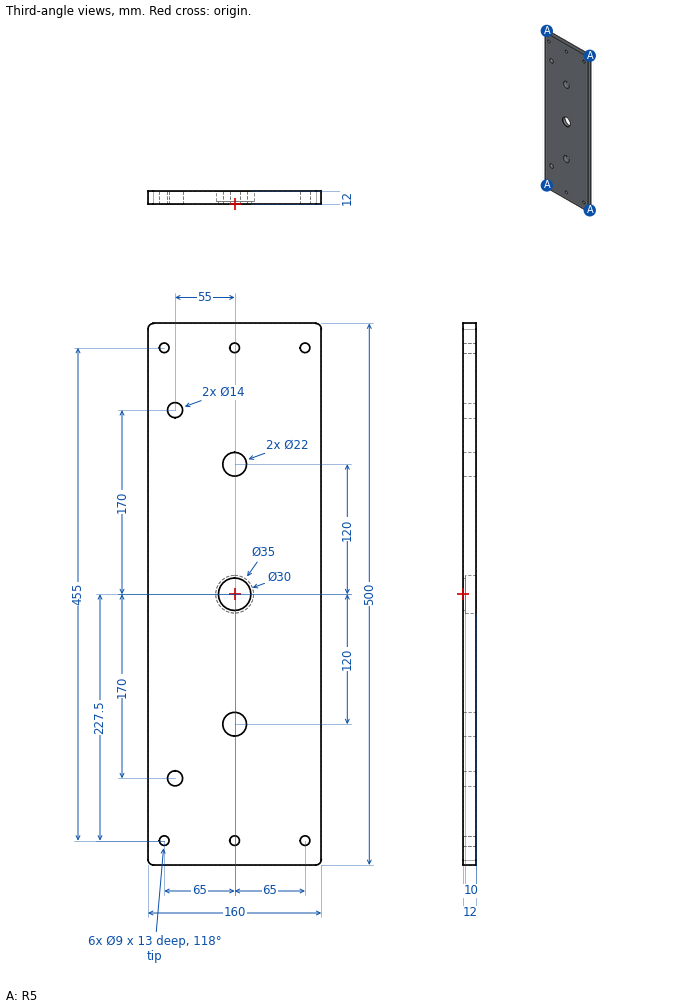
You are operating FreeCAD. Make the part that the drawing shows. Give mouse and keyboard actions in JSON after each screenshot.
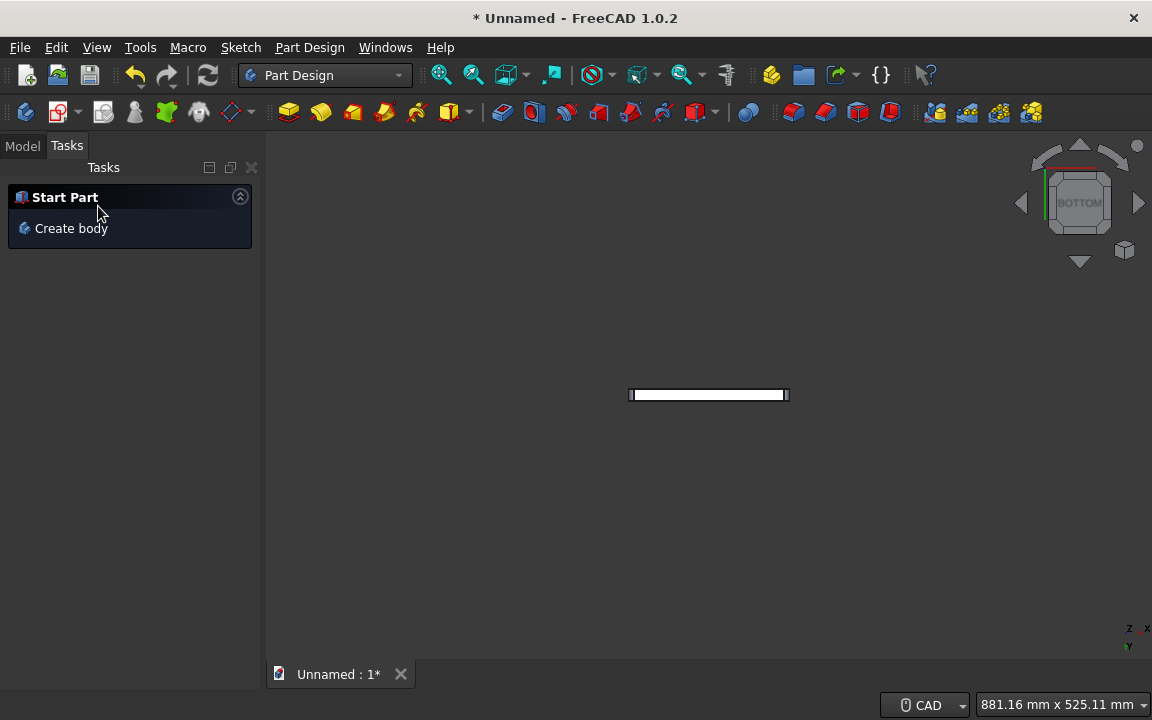
{"action": "left_click", "coordinate": [442, 76]}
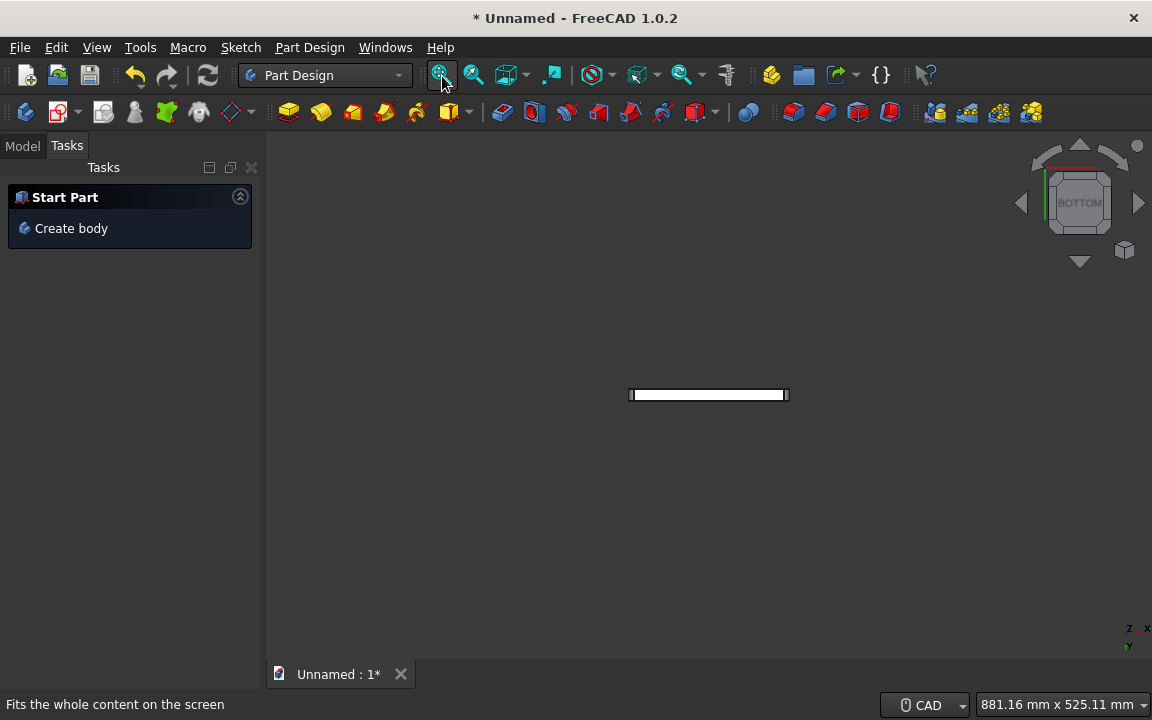
{"action": "left_click", "coordinate": [58, 112]}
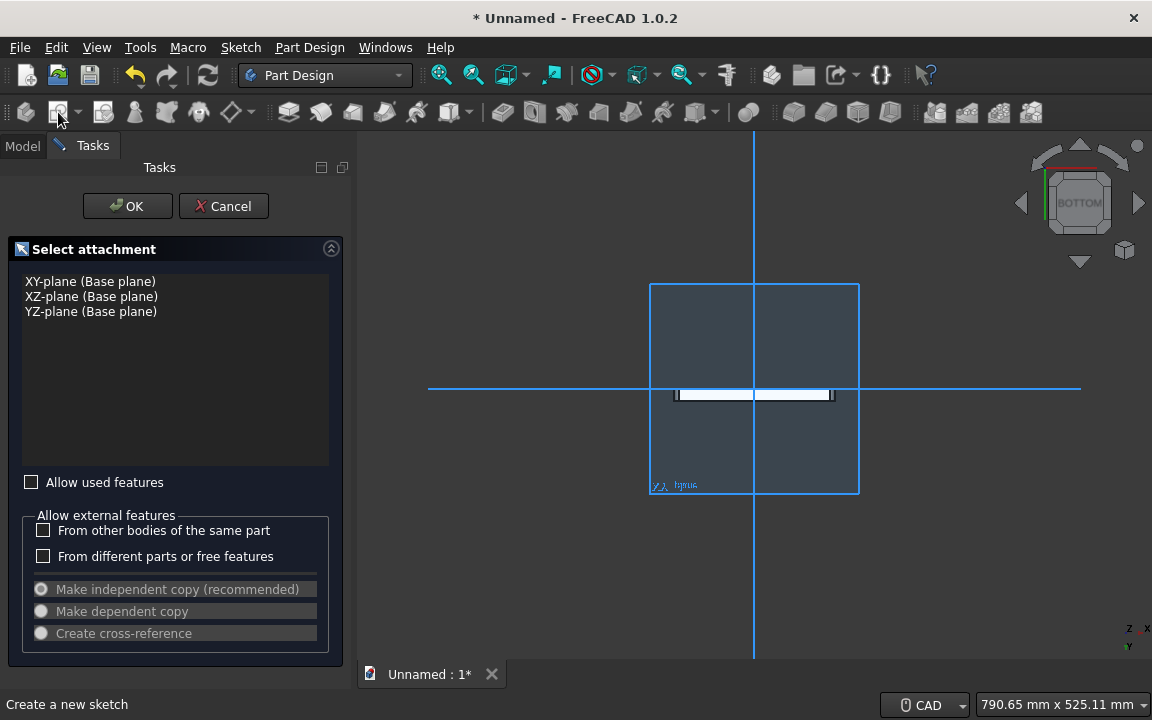
{"action": "left_click", "coordinate": [82, 296]}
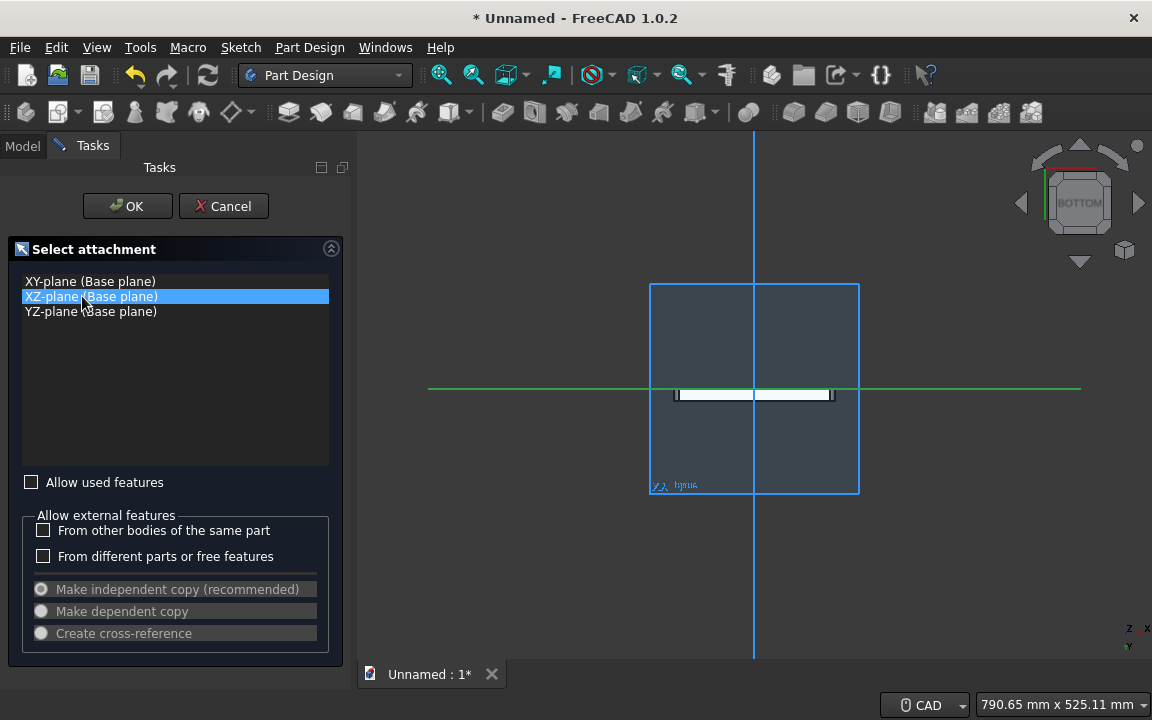
{"action": "left_click", "coordinate": [128, 206]}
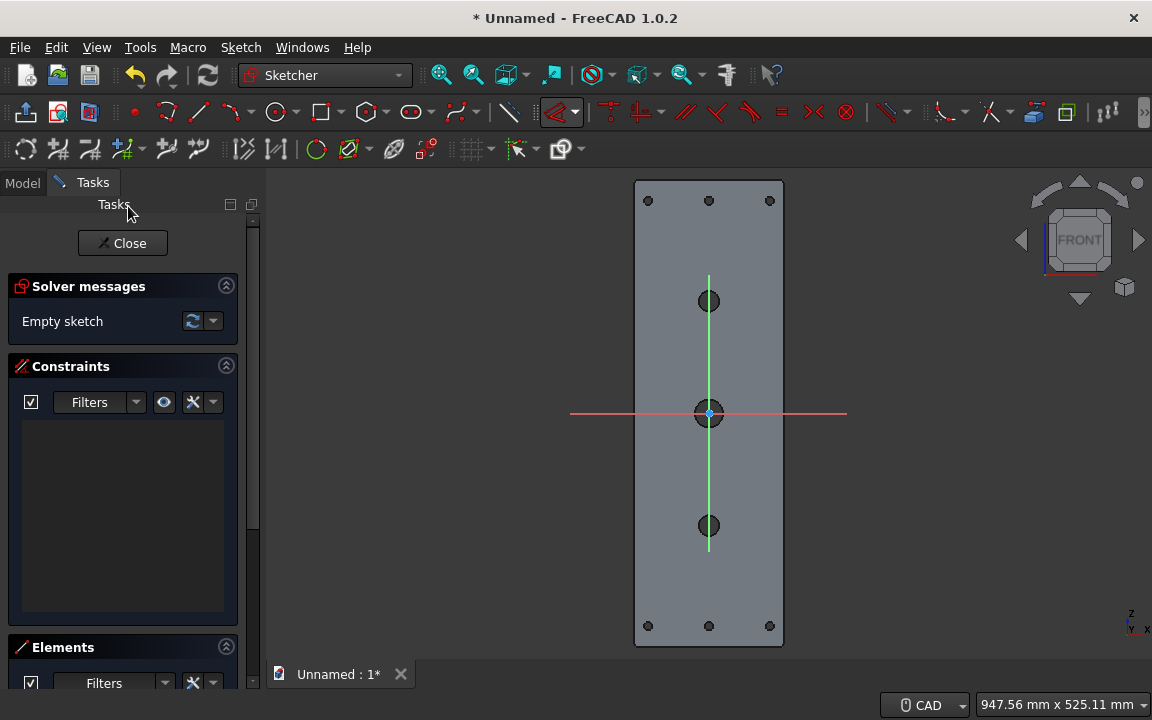
{"action": "left_click", "coordinate": [276, 112]}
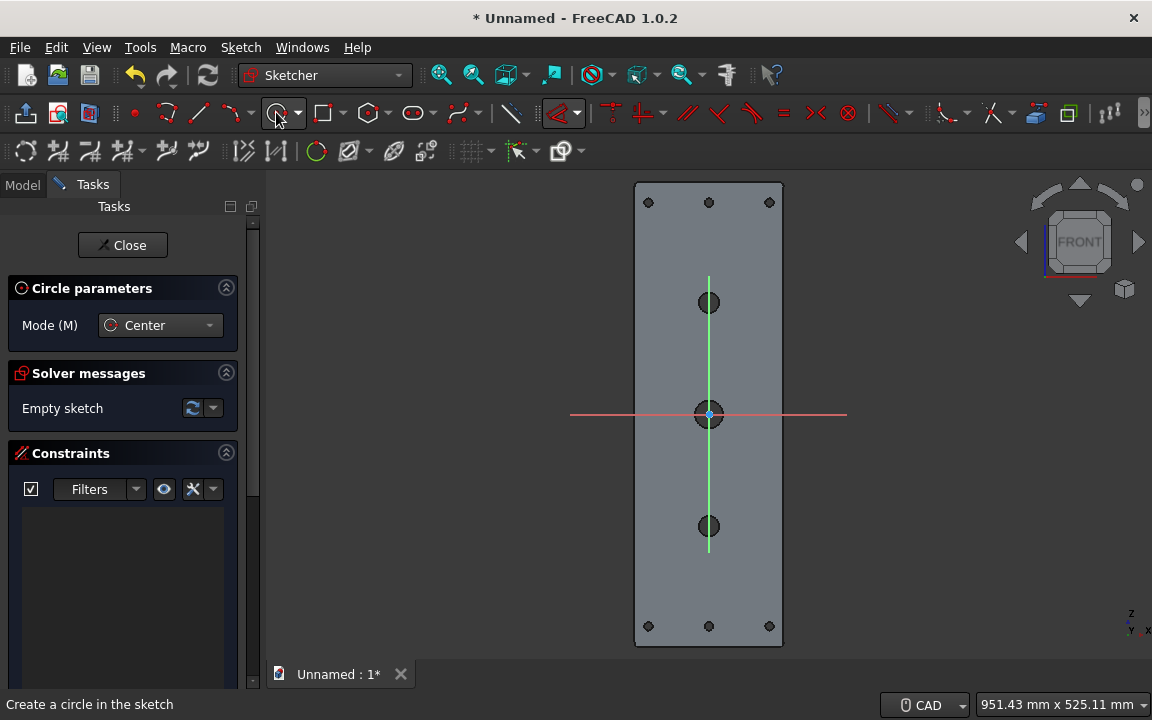
{"action": "scroll", "coordinate": [658, 256], "scroll_direction": "up", "scroll_amount": 7}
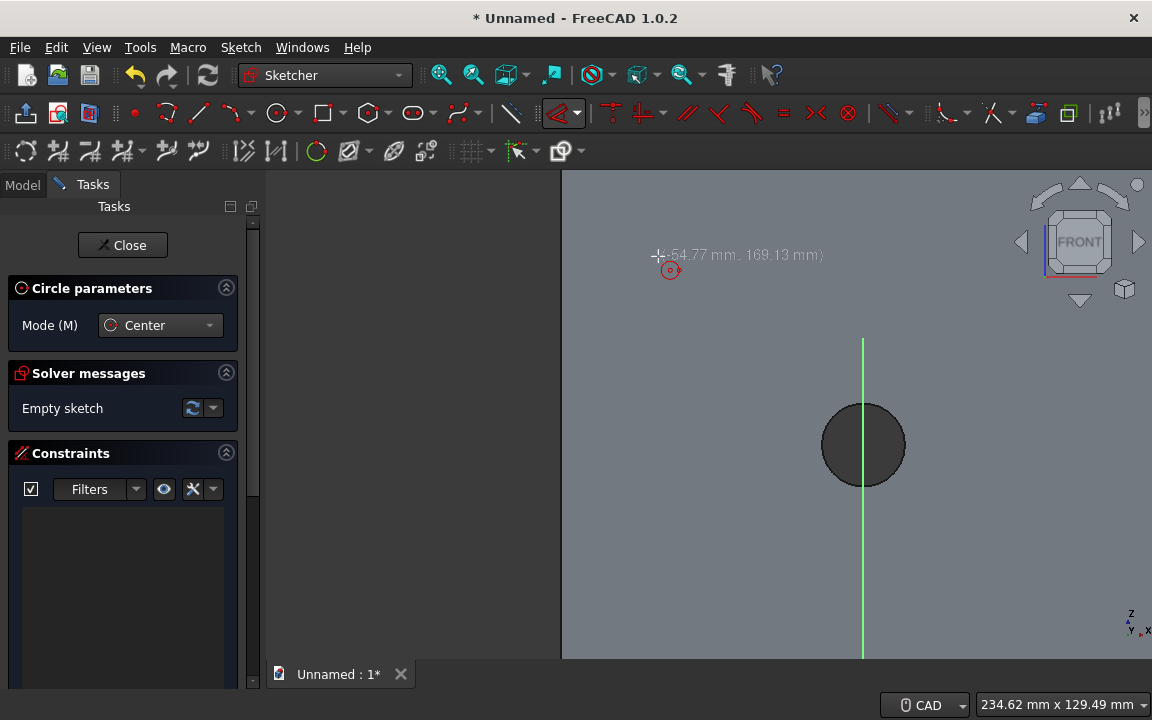
{"action": "scroll", "coordinate": [606, 256], "scroll_direction": "down", "scroll_amount": 7}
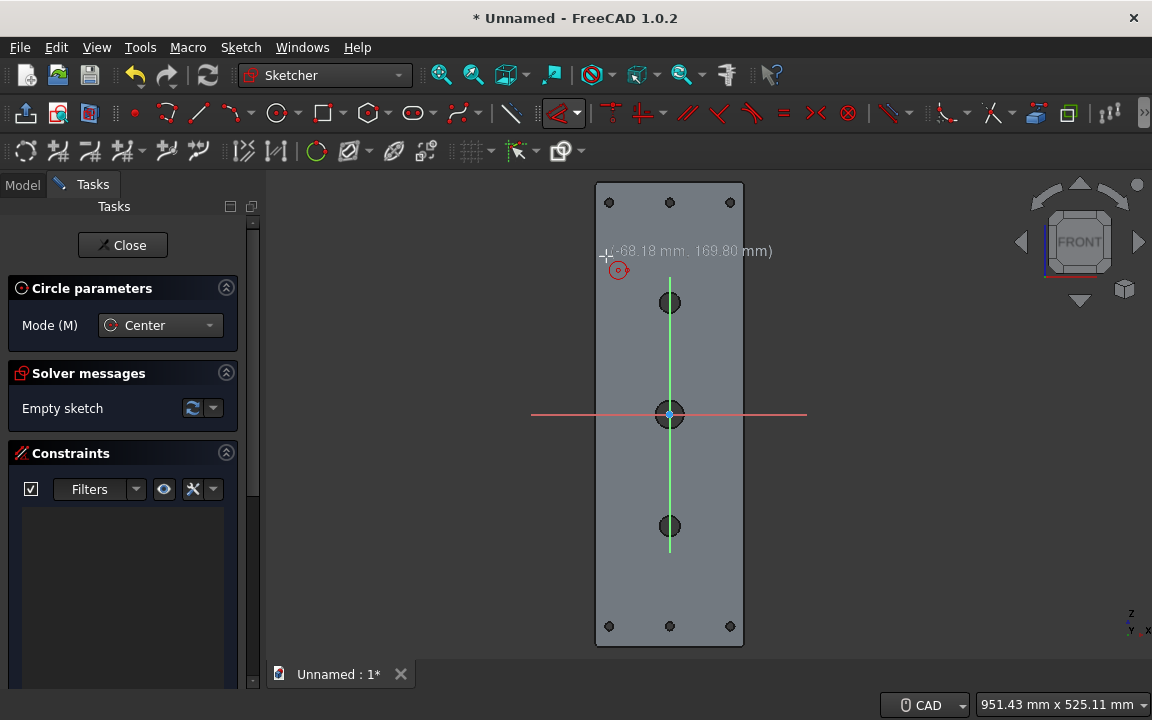
{"action": "left_click", "coordinate": [619, 256]}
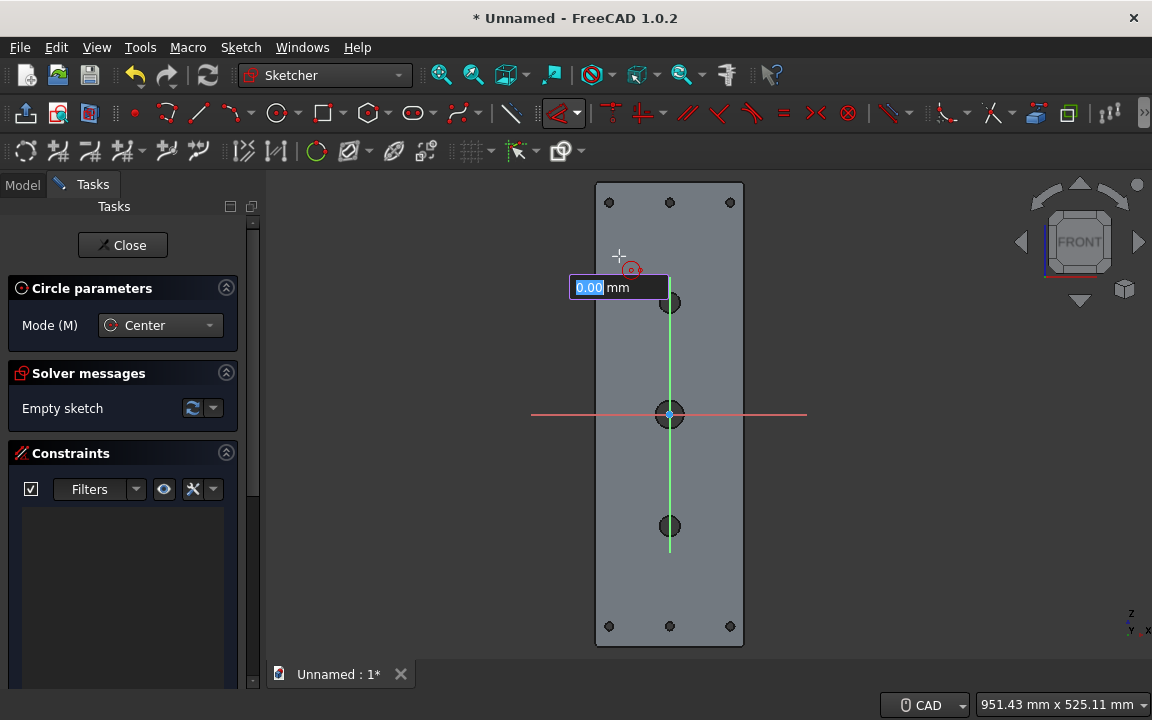
{"action": "scroll", "coordinate": [623, 252], "scroll_direction": "up", "scroll_amount": 5}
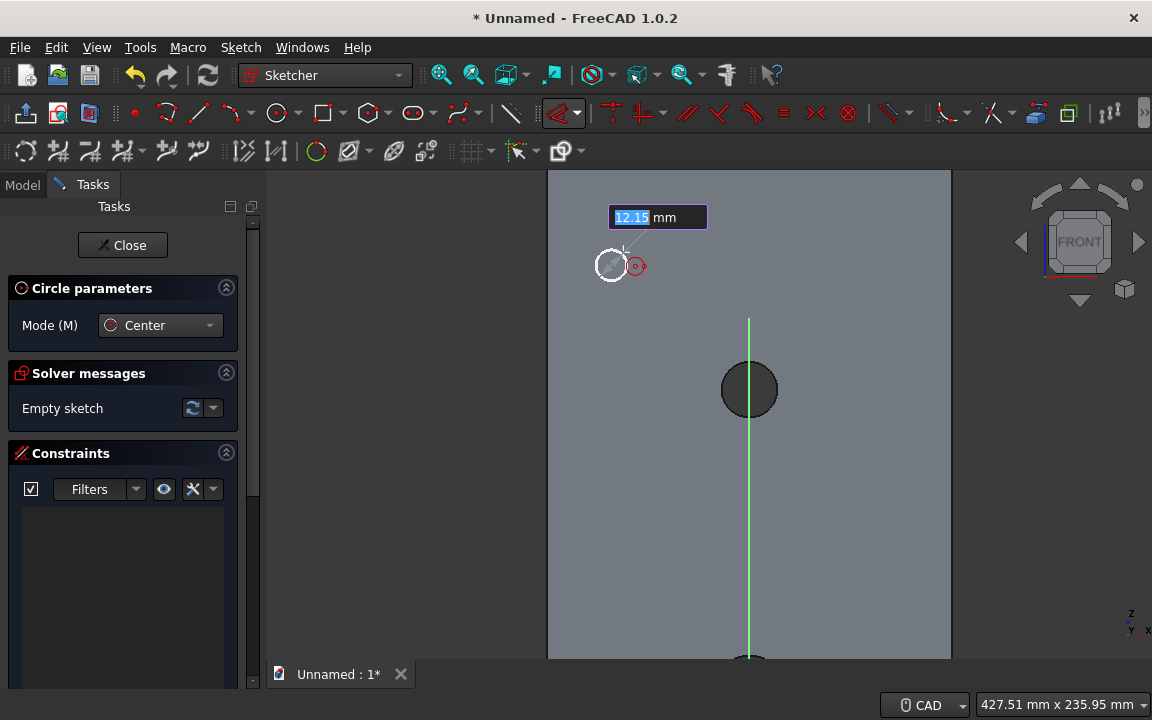
{"action": "left_click", "coordinate": [623, 251]}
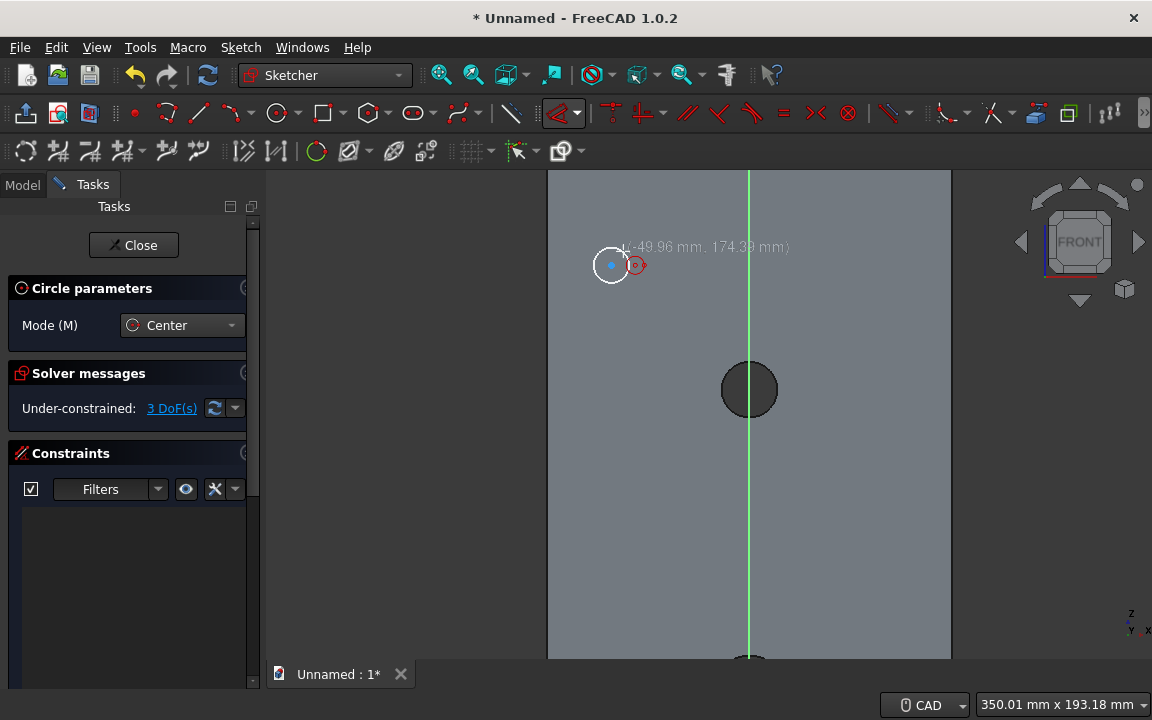
{"action": "scroll", "coordinate": [623, 252], "scroll_direction": "down", "scroll_amount": 5}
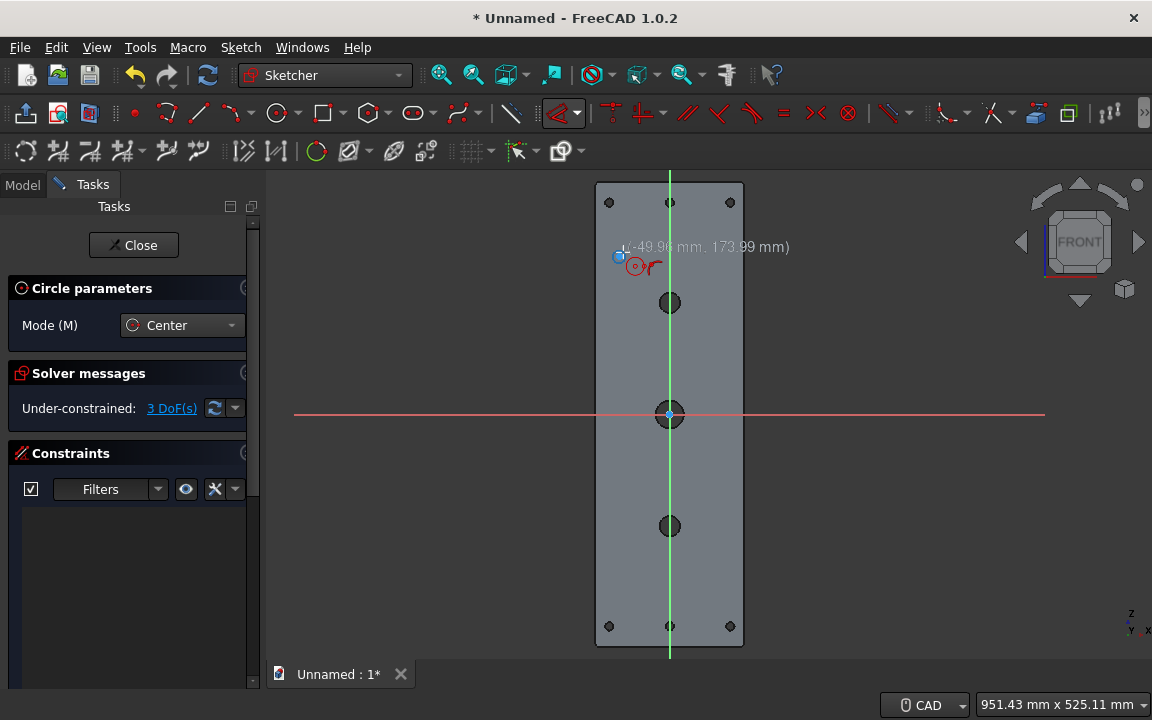
{"action": "scroll", "coordinate": [619, 573], "scroll_direction": "up", "scroll_amount": 7}